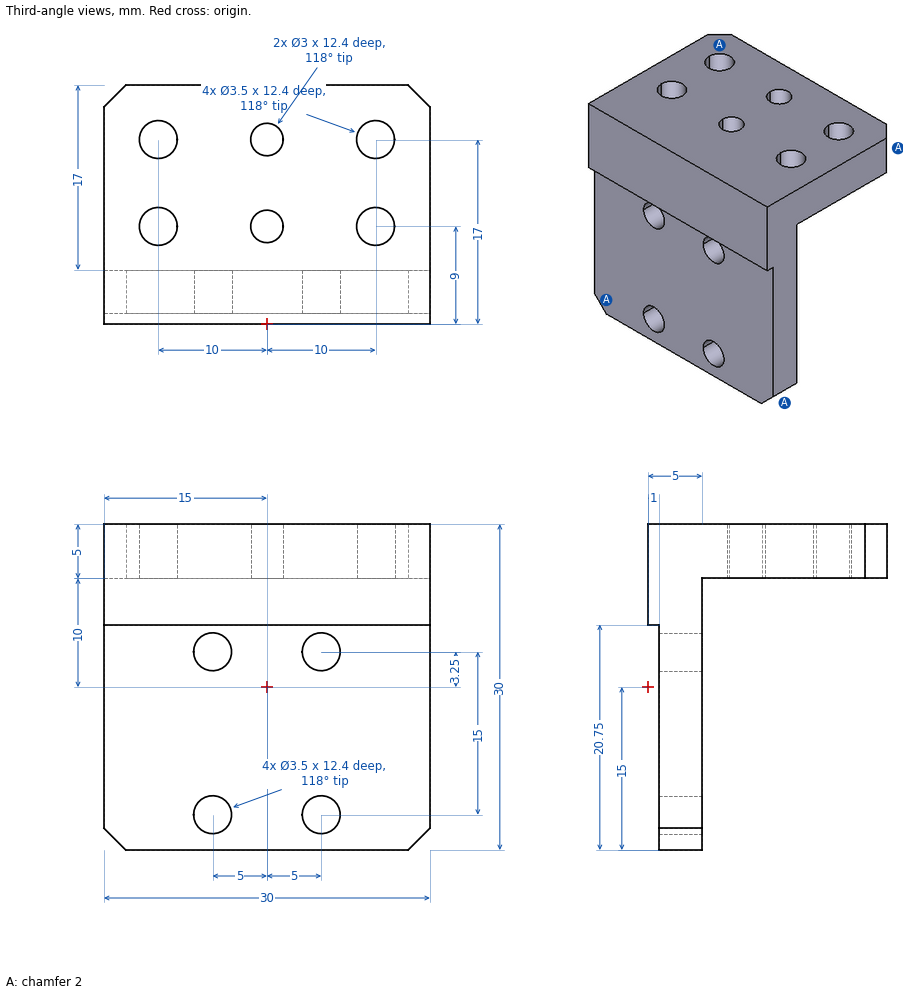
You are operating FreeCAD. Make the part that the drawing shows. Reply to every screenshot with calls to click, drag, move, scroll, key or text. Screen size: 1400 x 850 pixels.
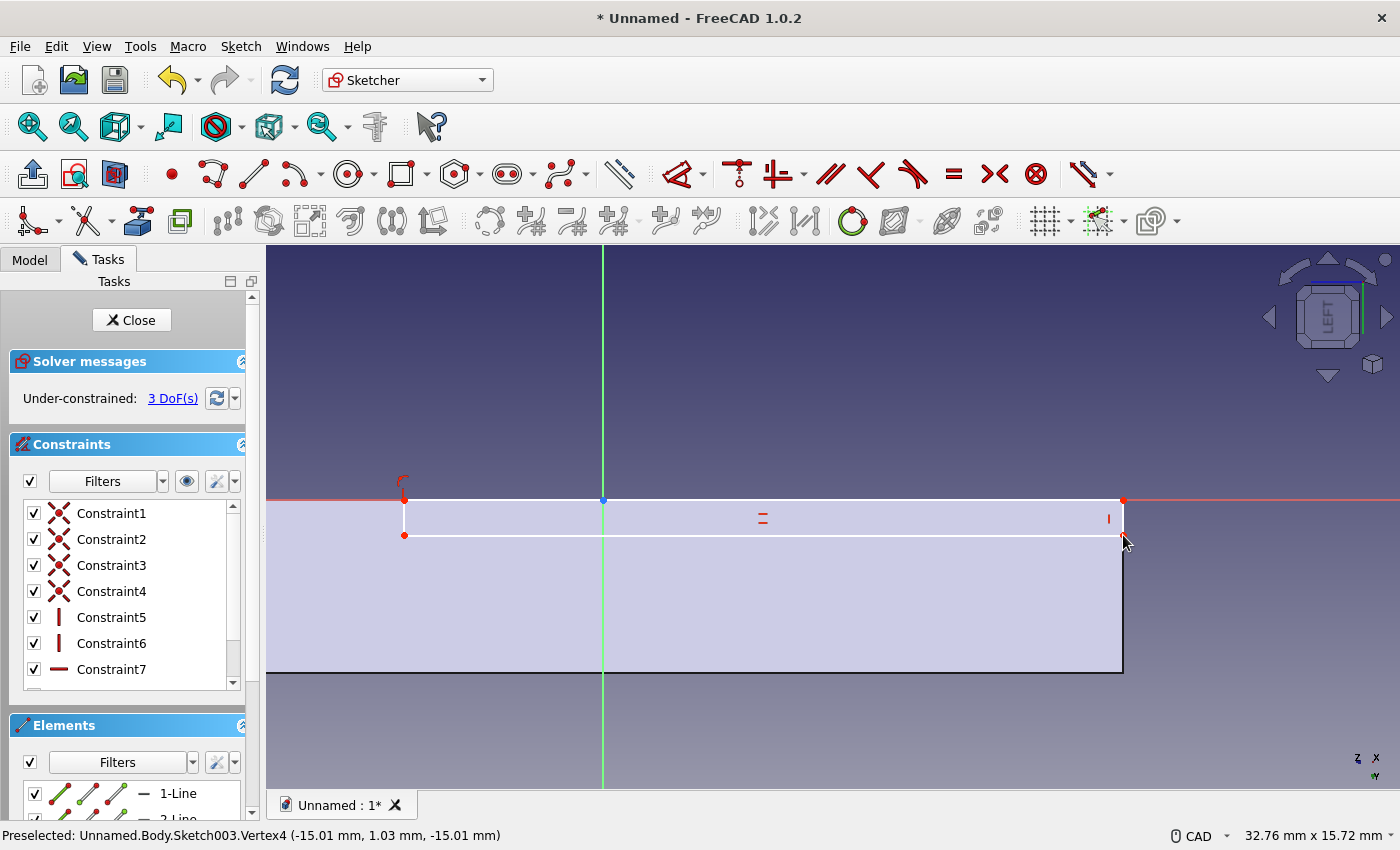
click(676, 174)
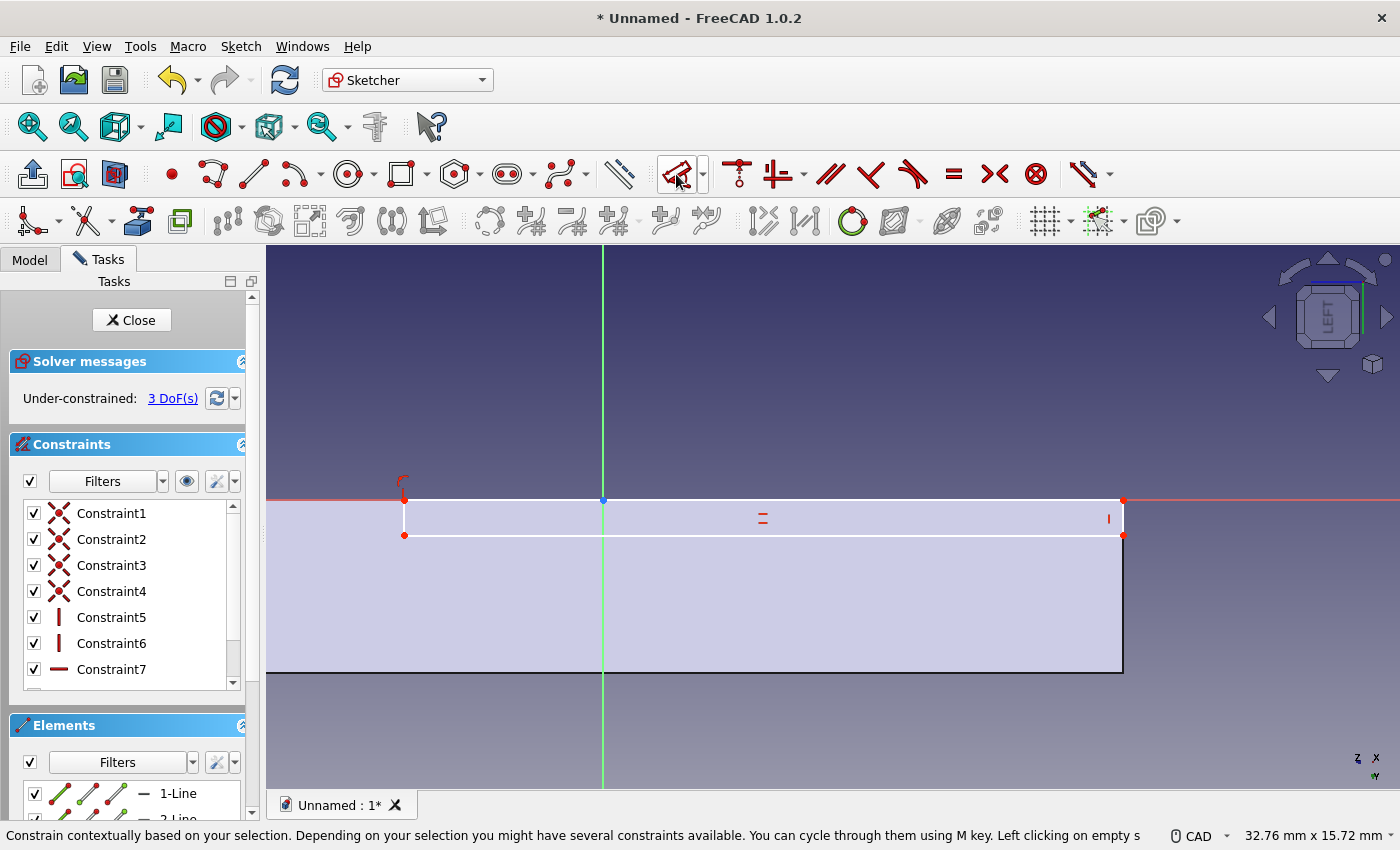
scroll(404, 511, up, 2)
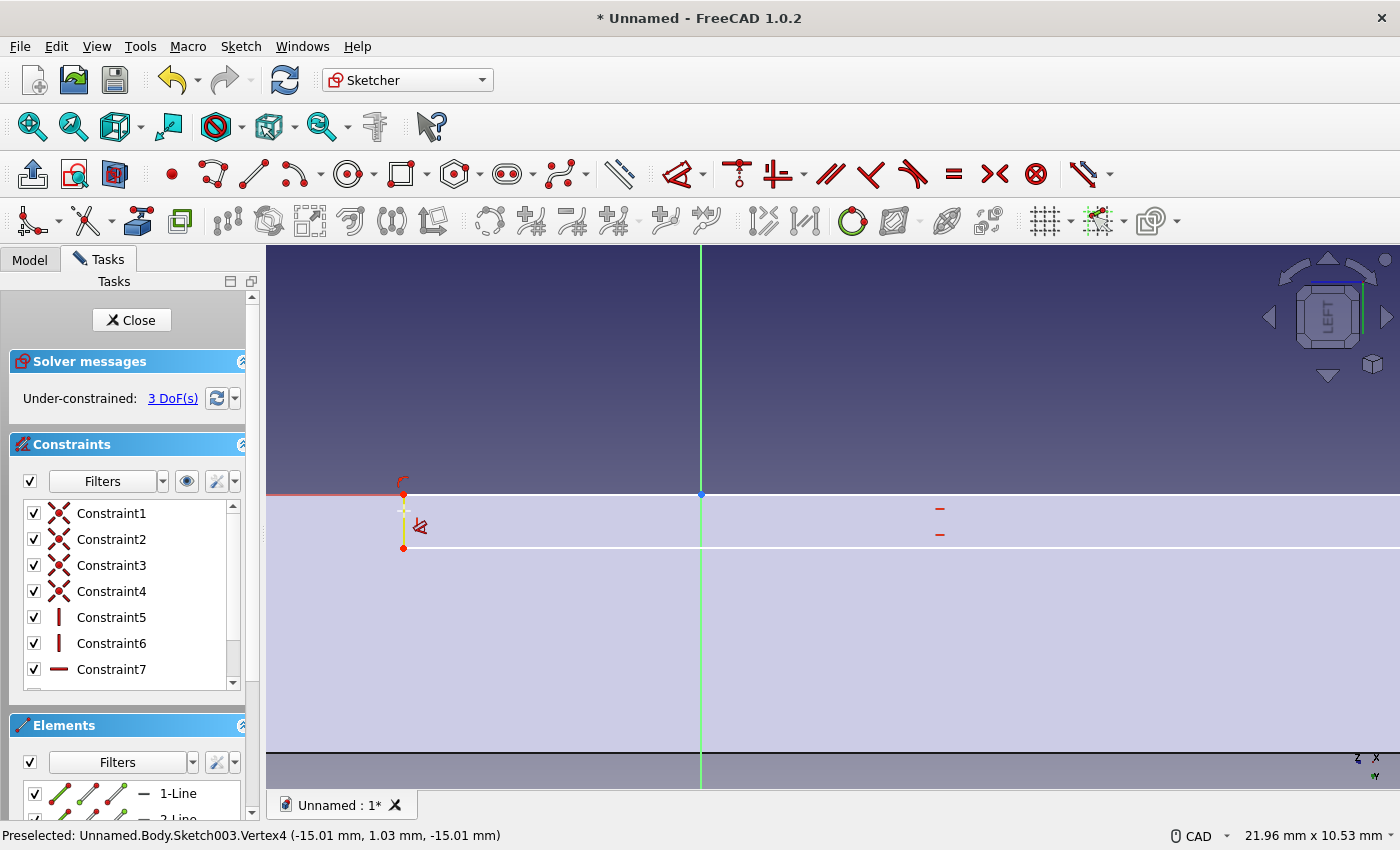
click(404, 511)
click(370, 521)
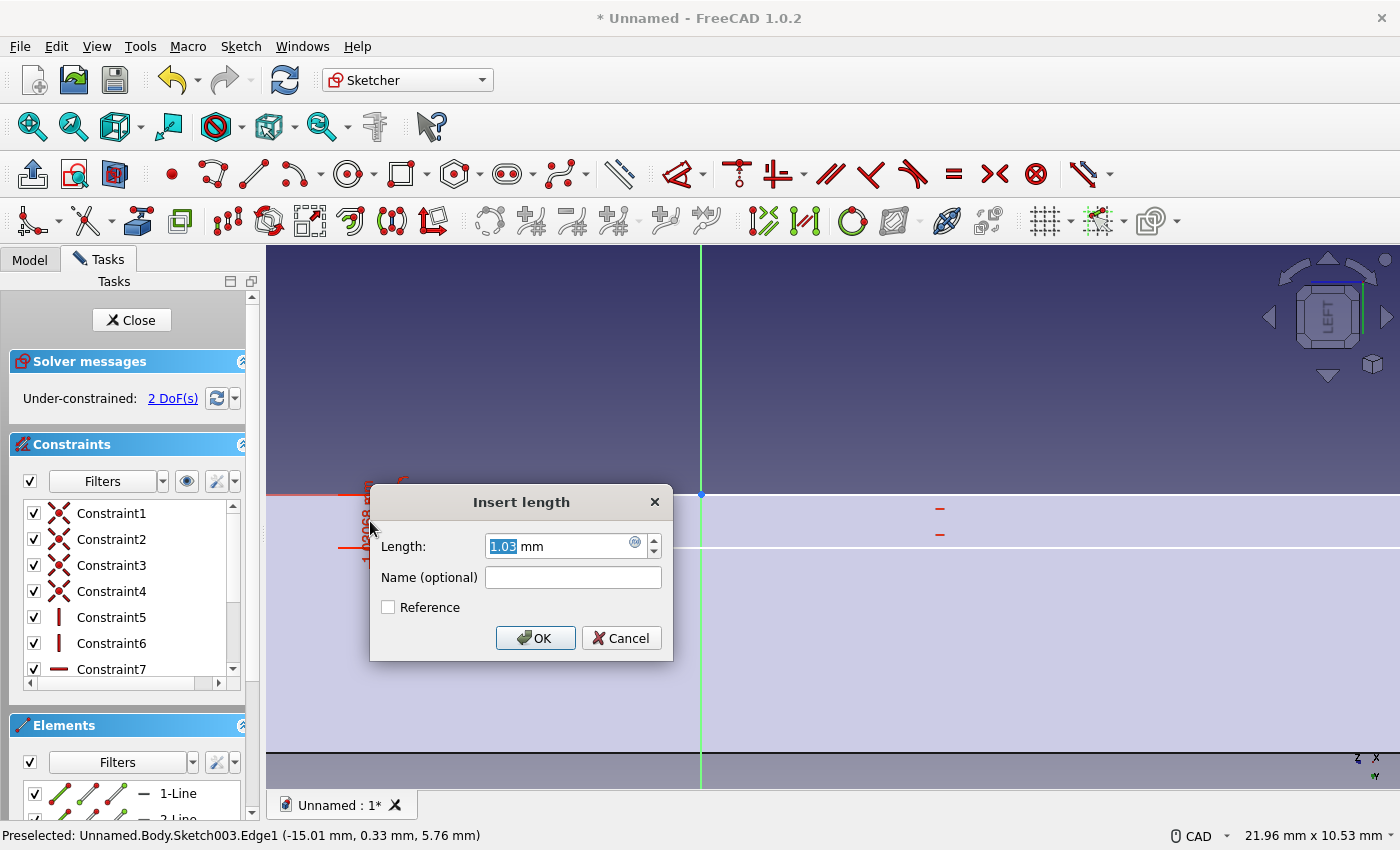
text(1)
key(Return)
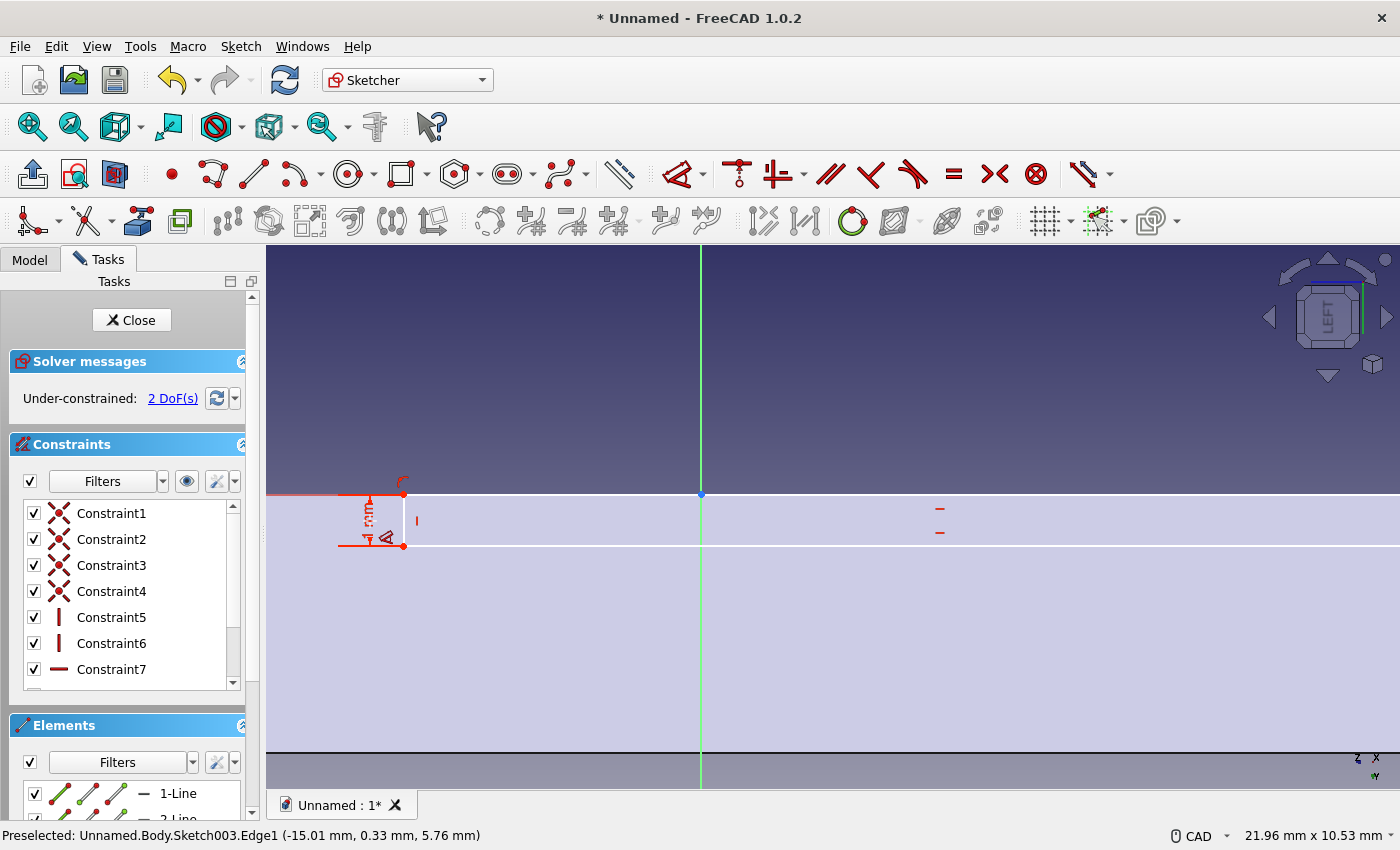
scroll(407, 510, down, 2)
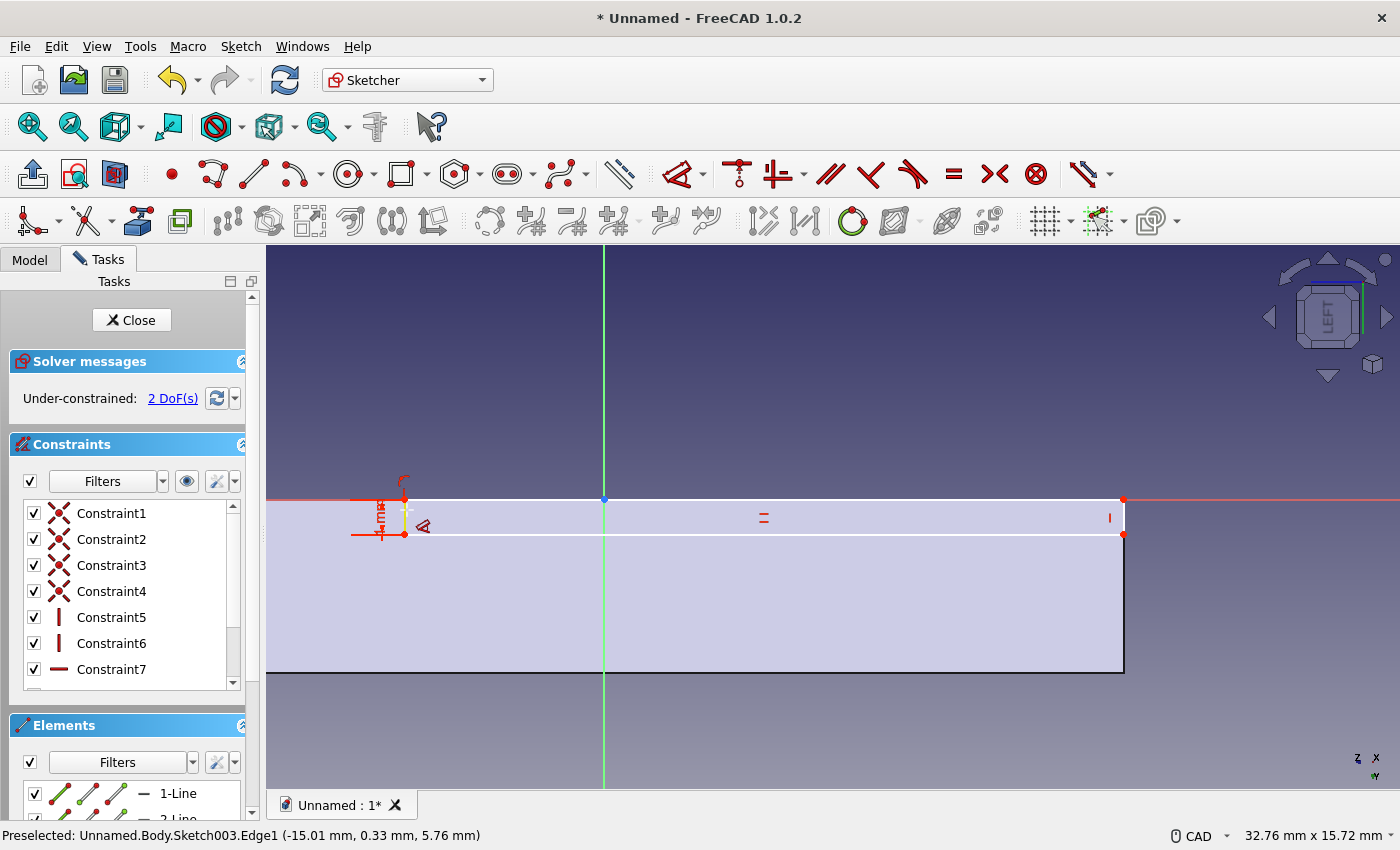
click(1124, 535)
click(864, 569)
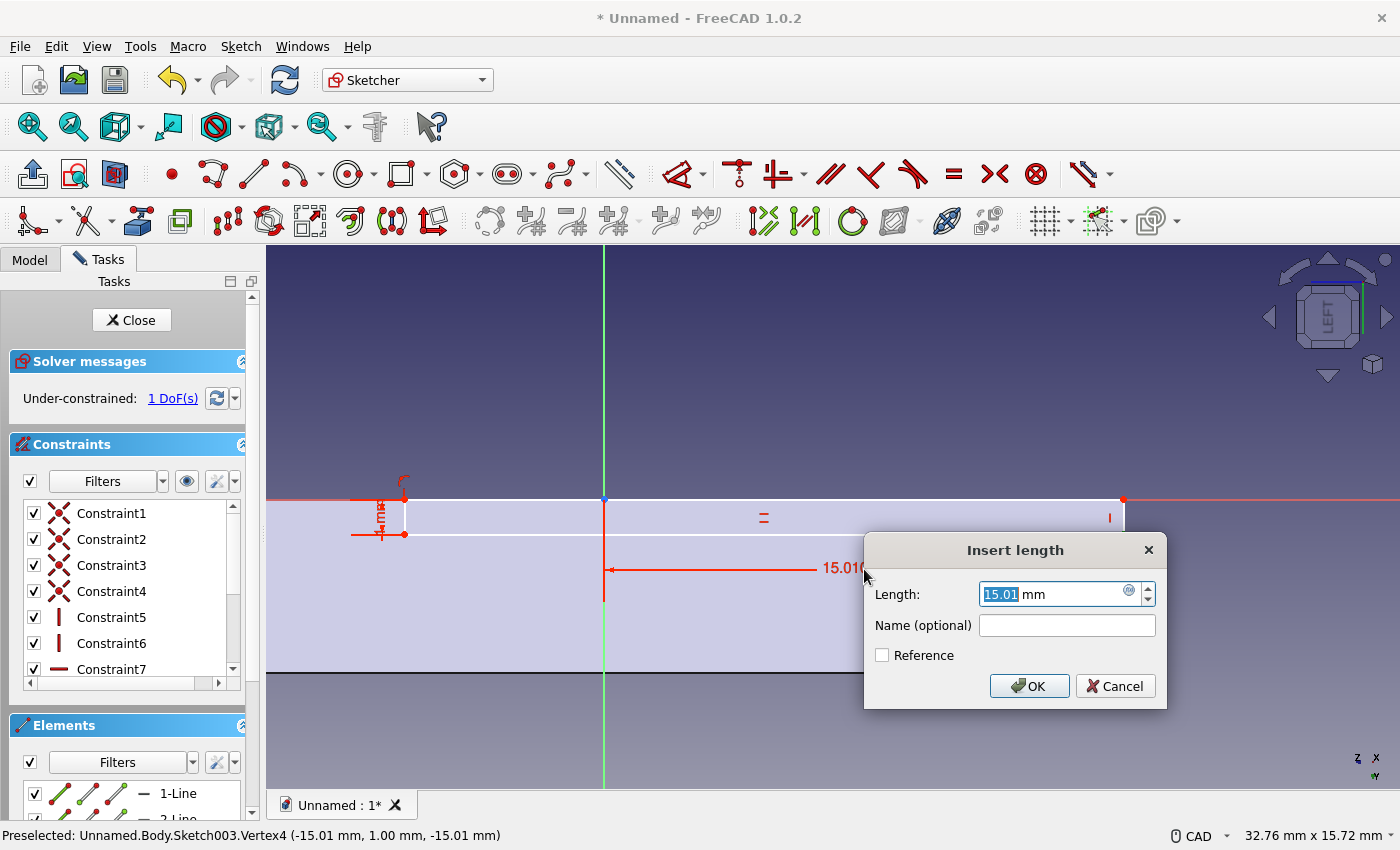
text(15)
key(Return)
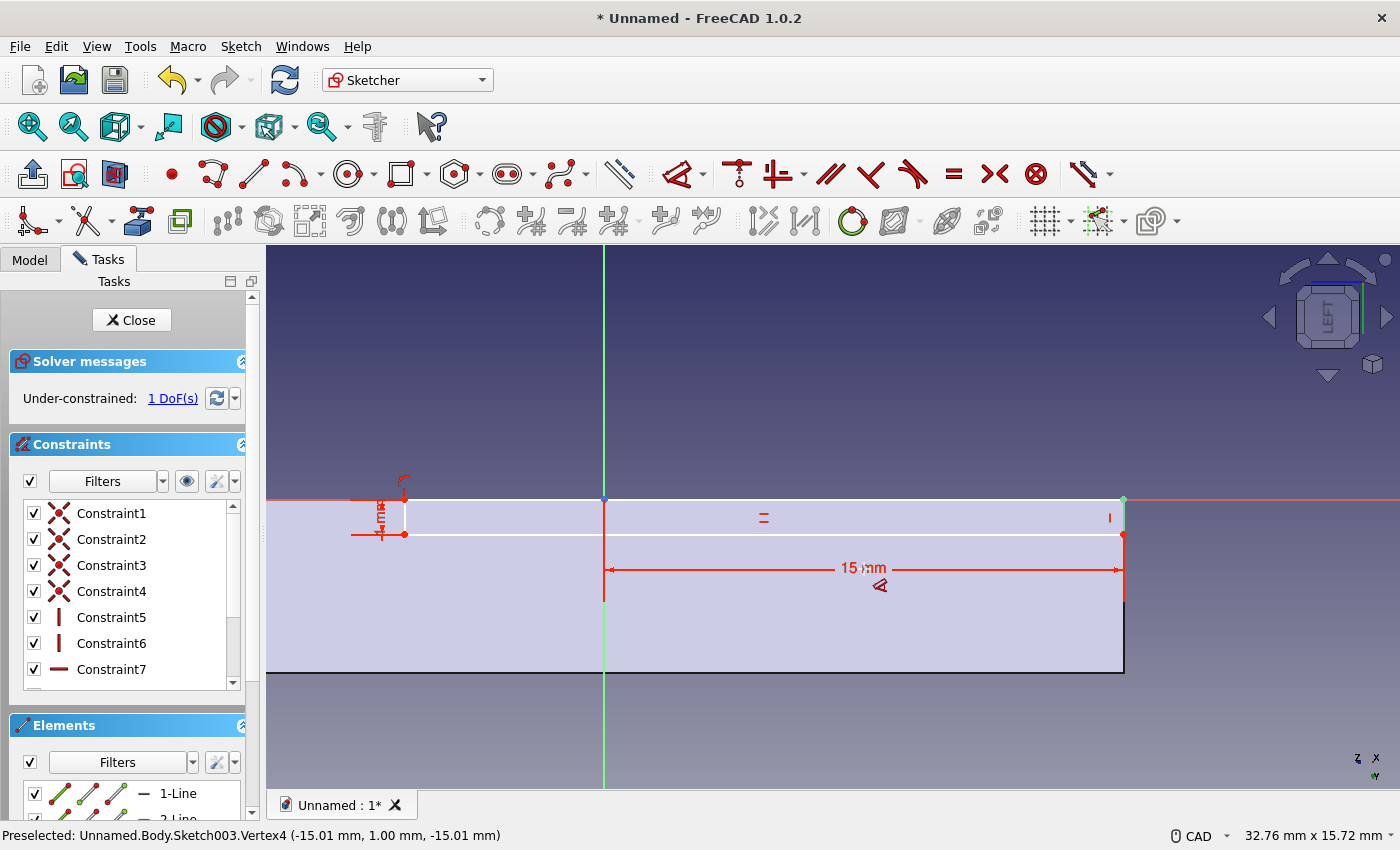
click(621, 535)
click(764, 569)